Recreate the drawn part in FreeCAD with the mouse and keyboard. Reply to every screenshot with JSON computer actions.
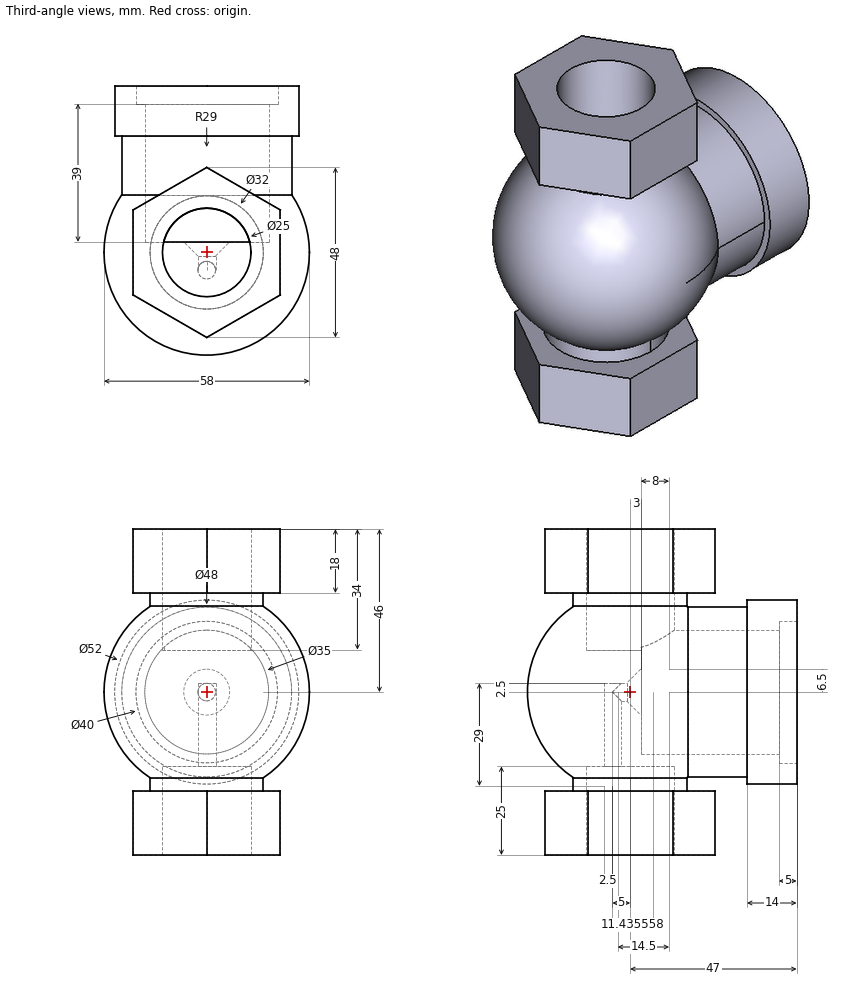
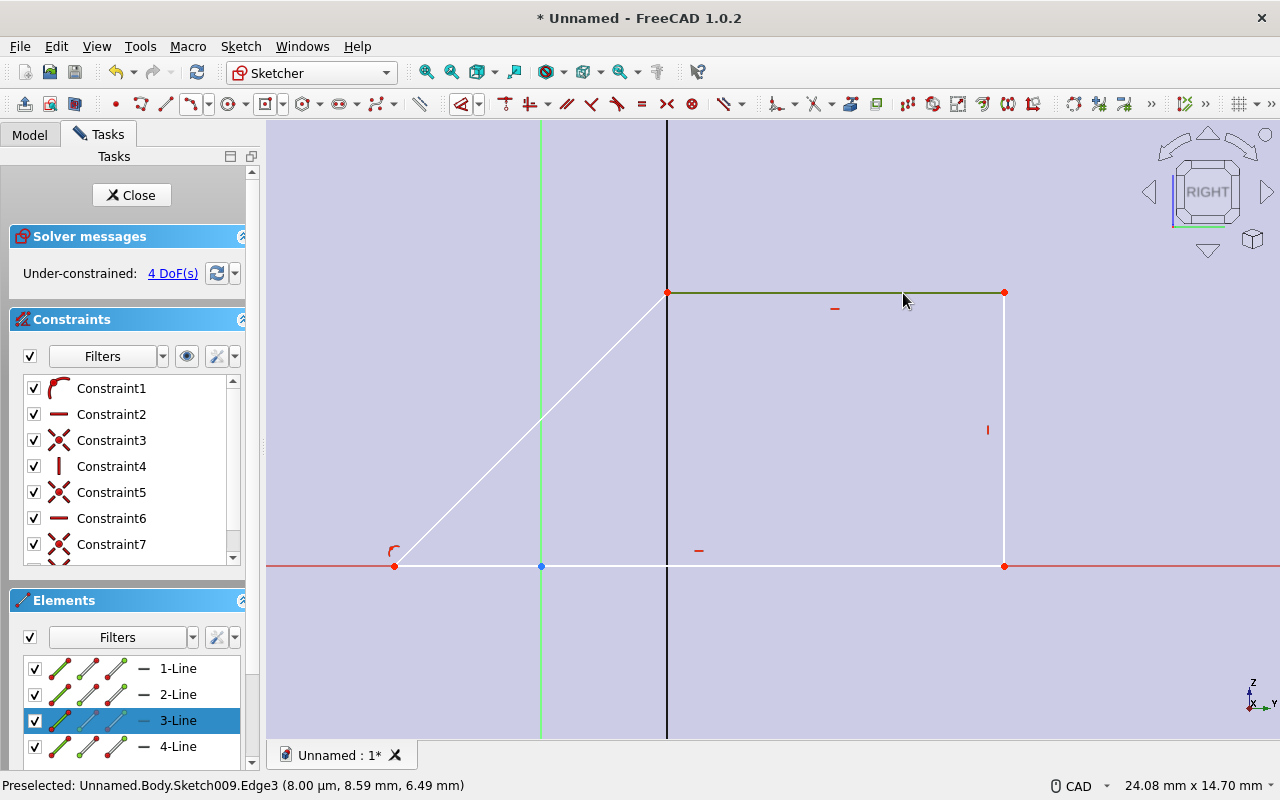
{"action": "left_click", "coordinate": [478, 104]}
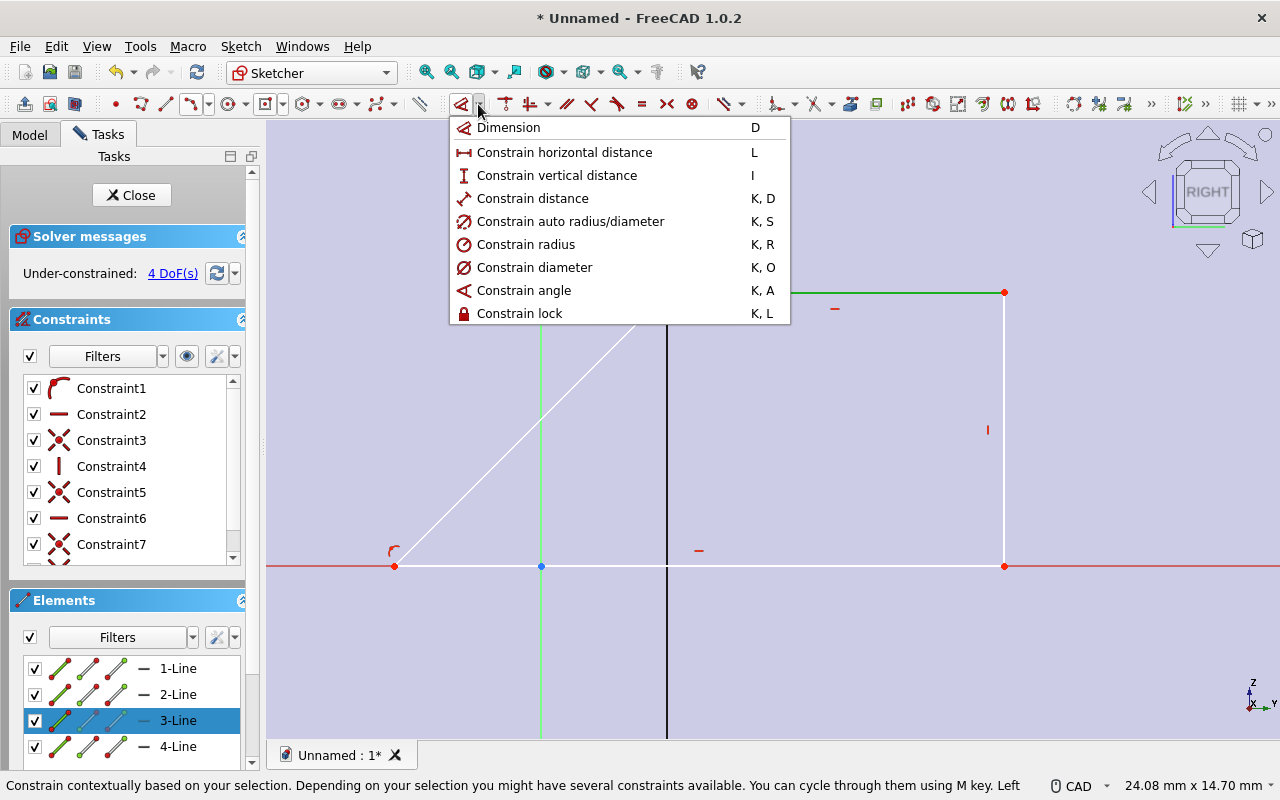
{"action": "left_click", "coordinate": [620, 152]}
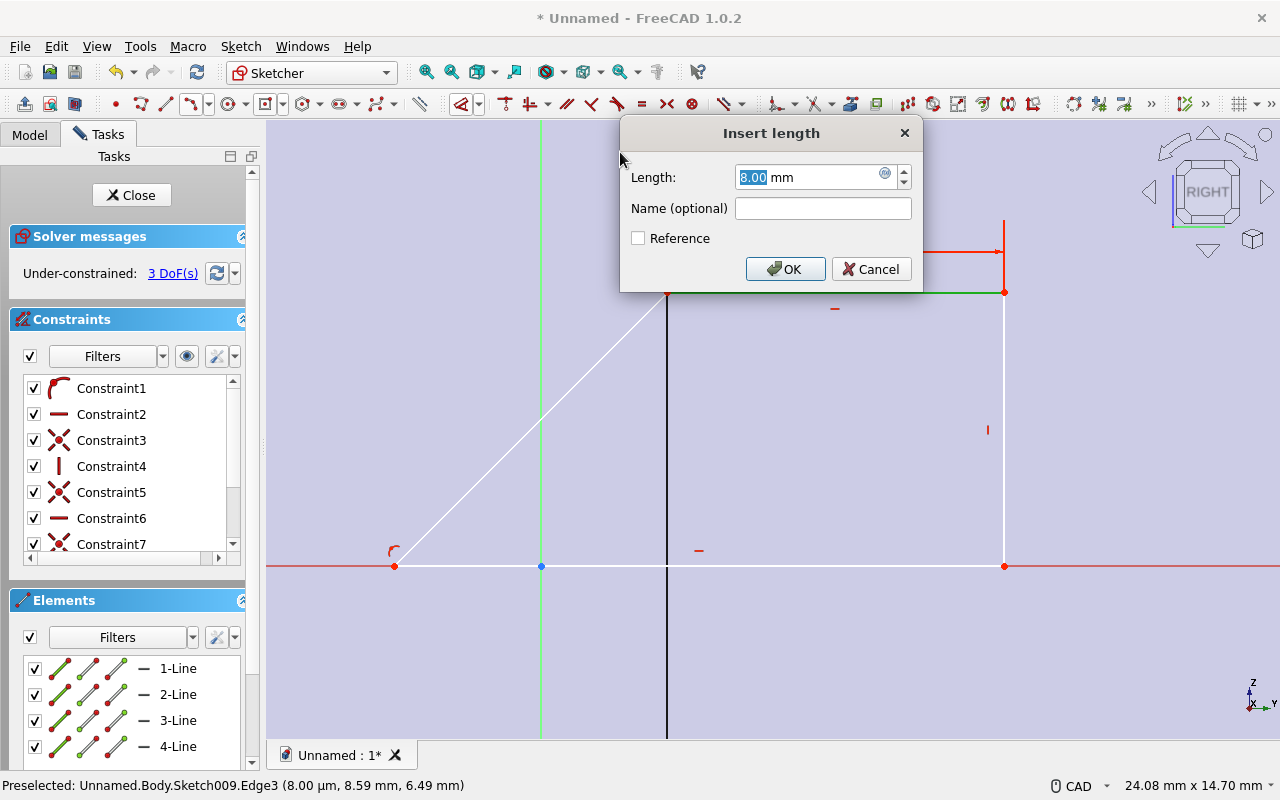
{"action": "type", "text": "8"}
{"action": "key", "text": "Return"}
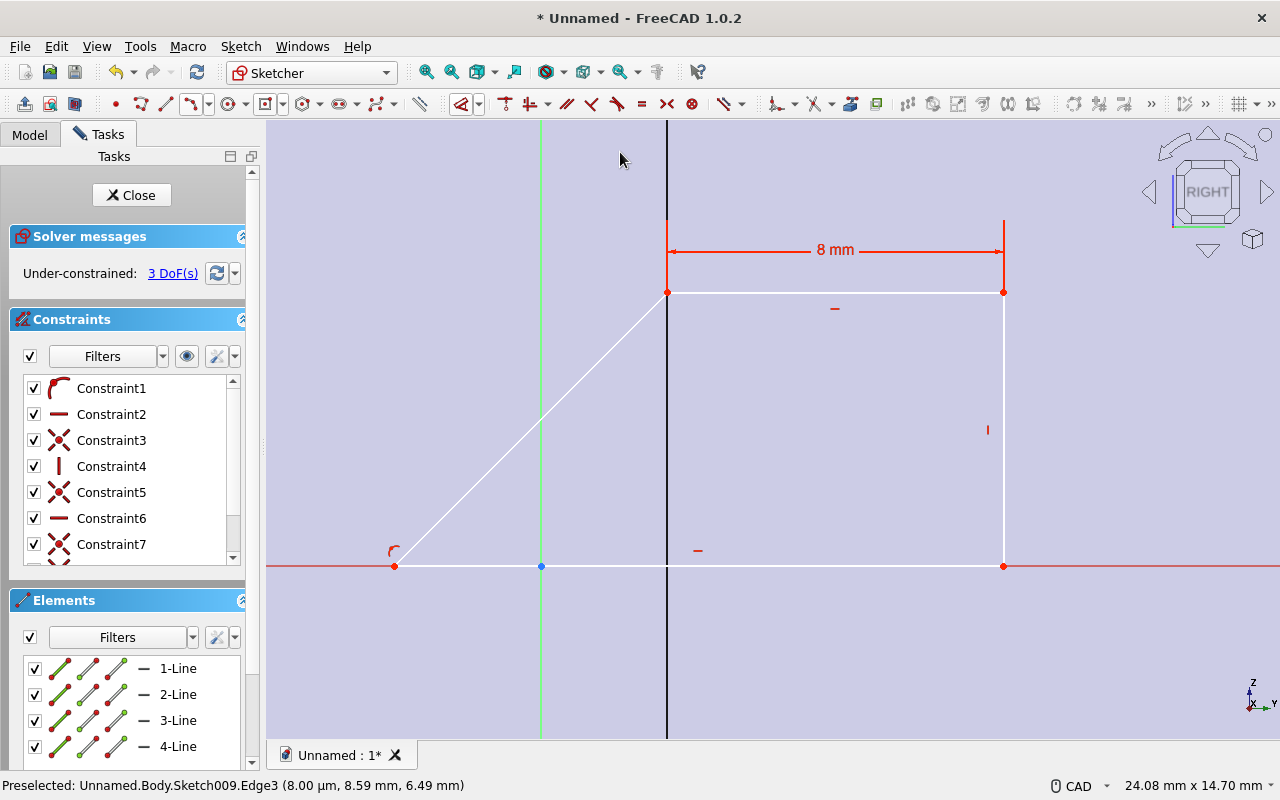
{"action": "left_click", "coordinate": [667, 293]}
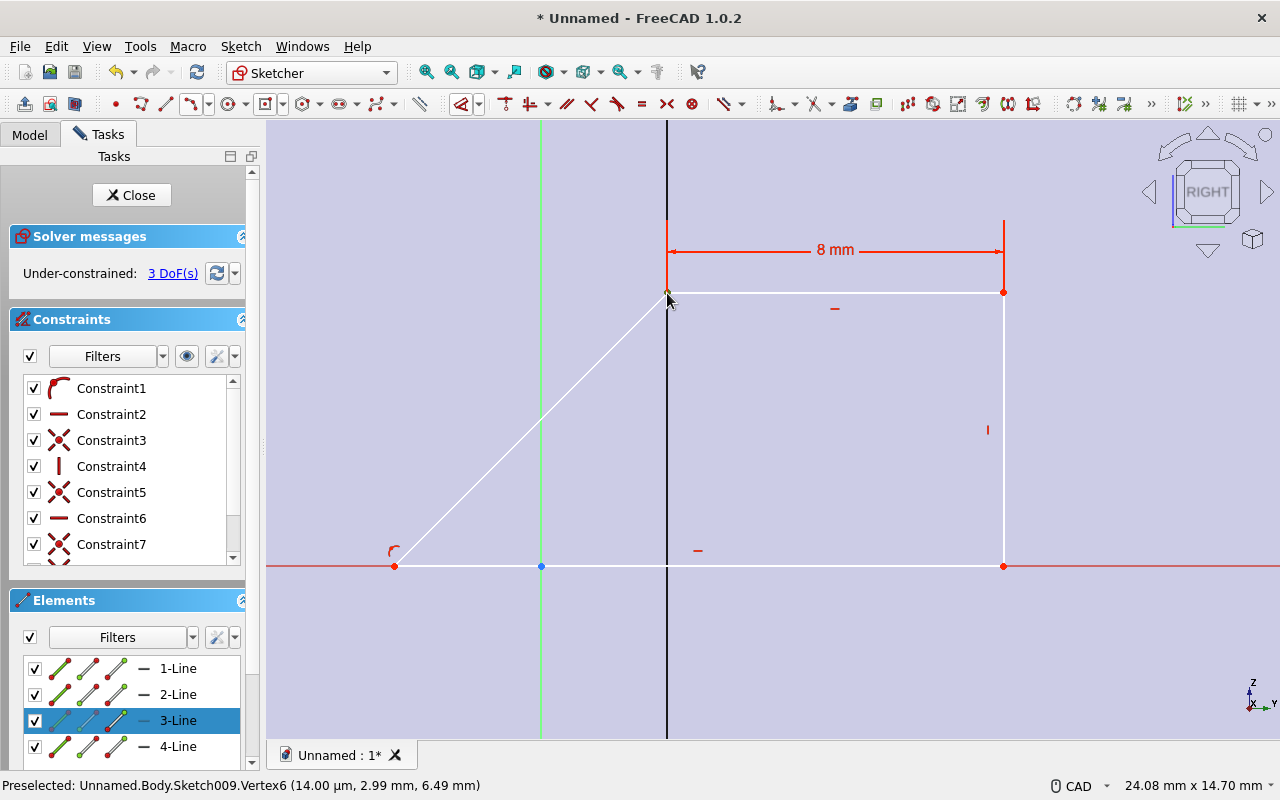
{"action": "key", "text": "l"}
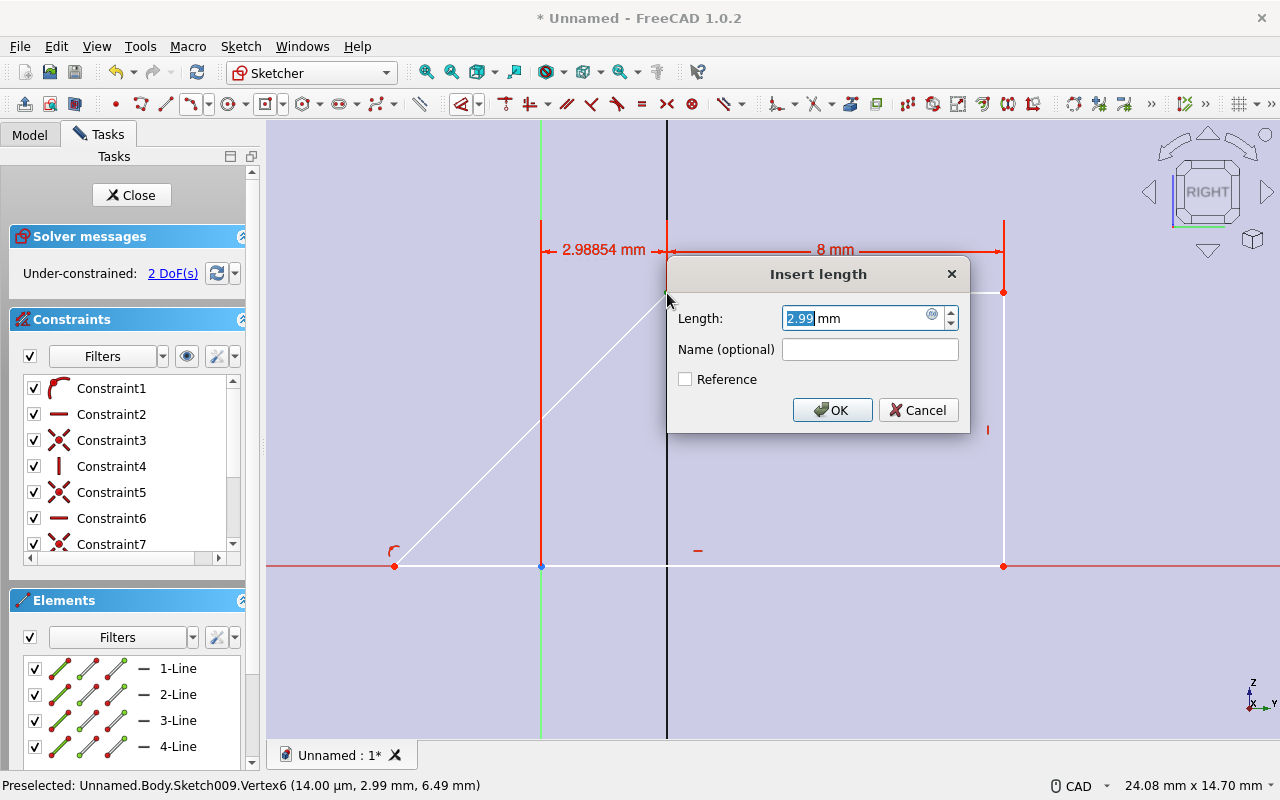
{"action": "type", "text": "3"}
{"action": "key", "text": "Return"}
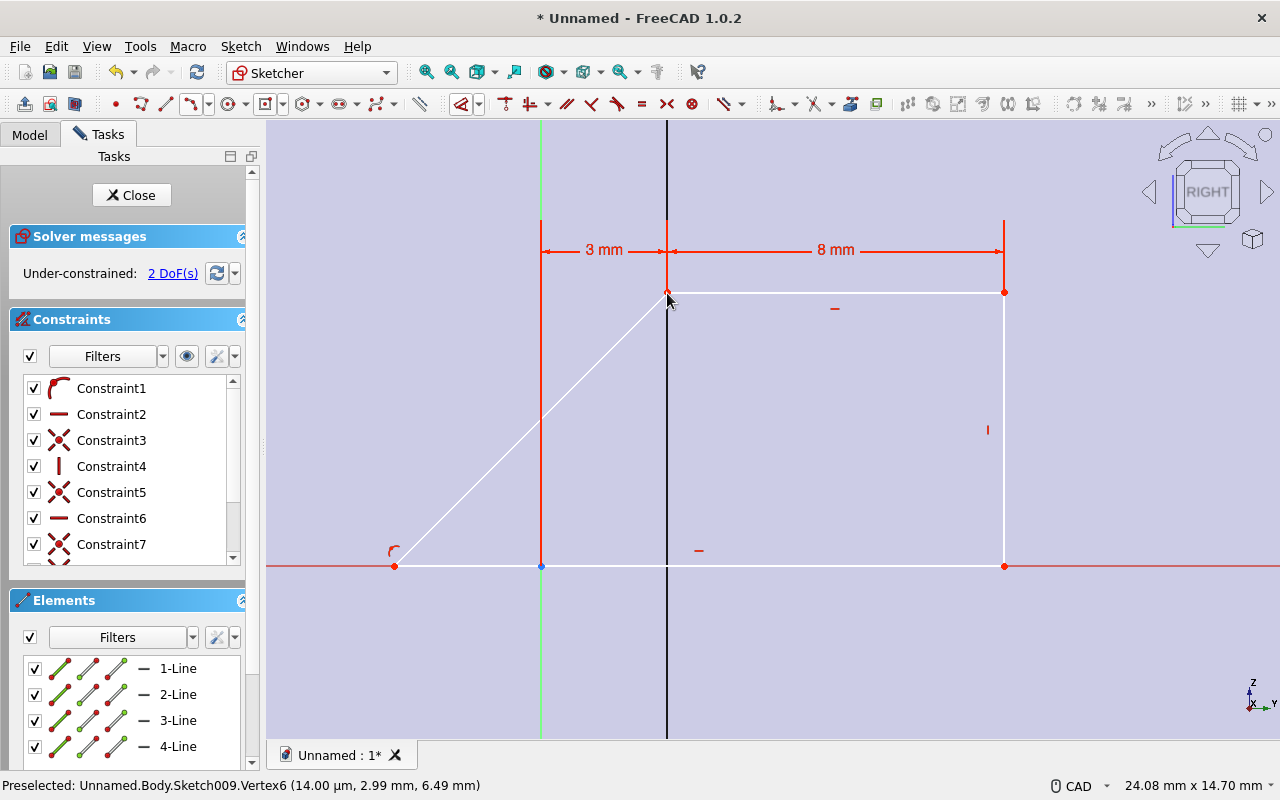
{"action": "left_click", "coordinate": [1004, 484]}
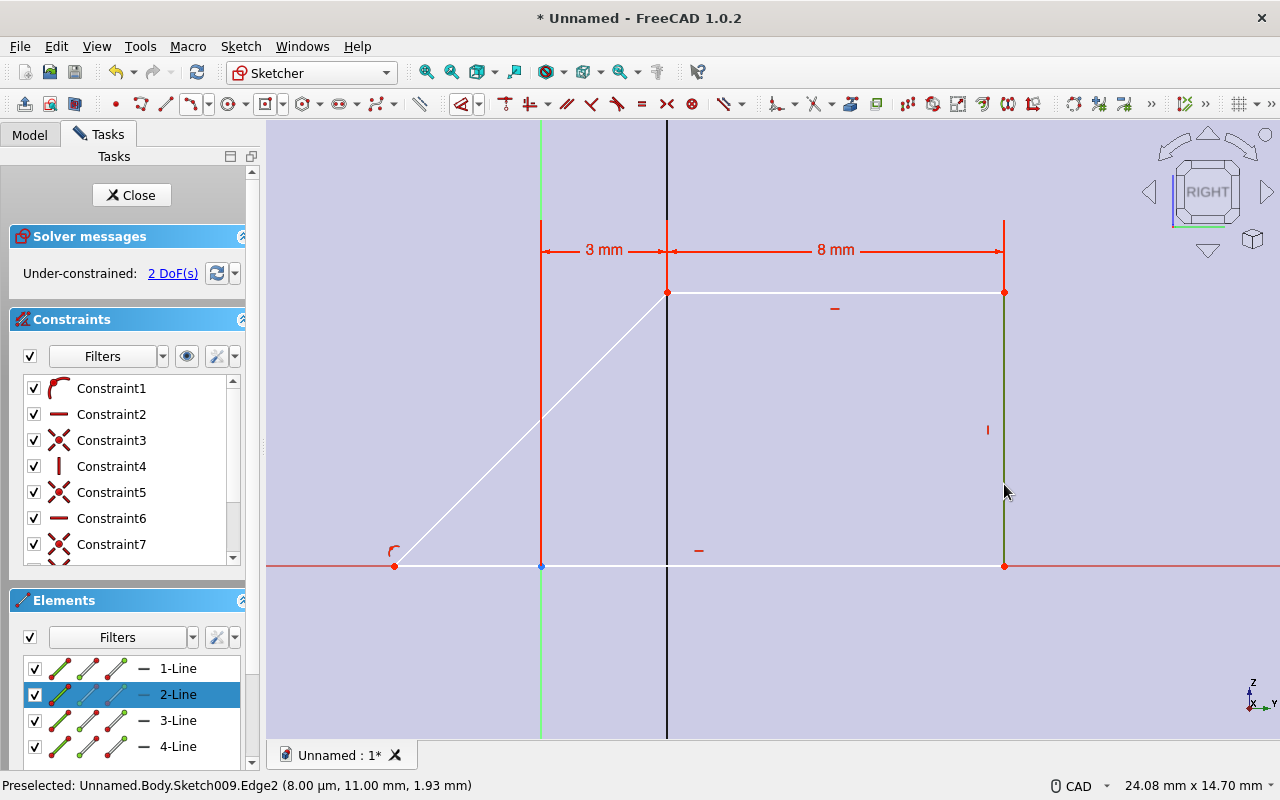
{"action": "key", "text": "i"}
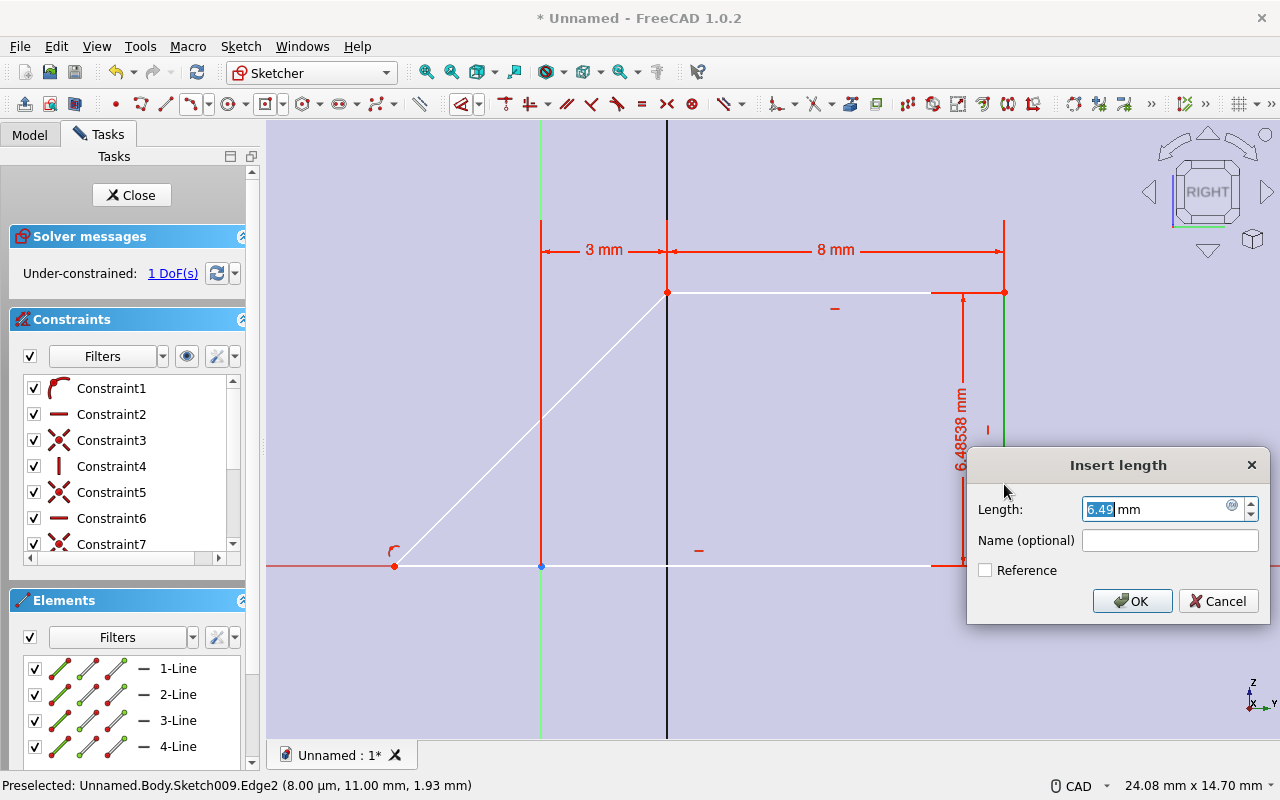
{"action": "type", "text": "6.5"}
{"action": "key", "text": "Return"}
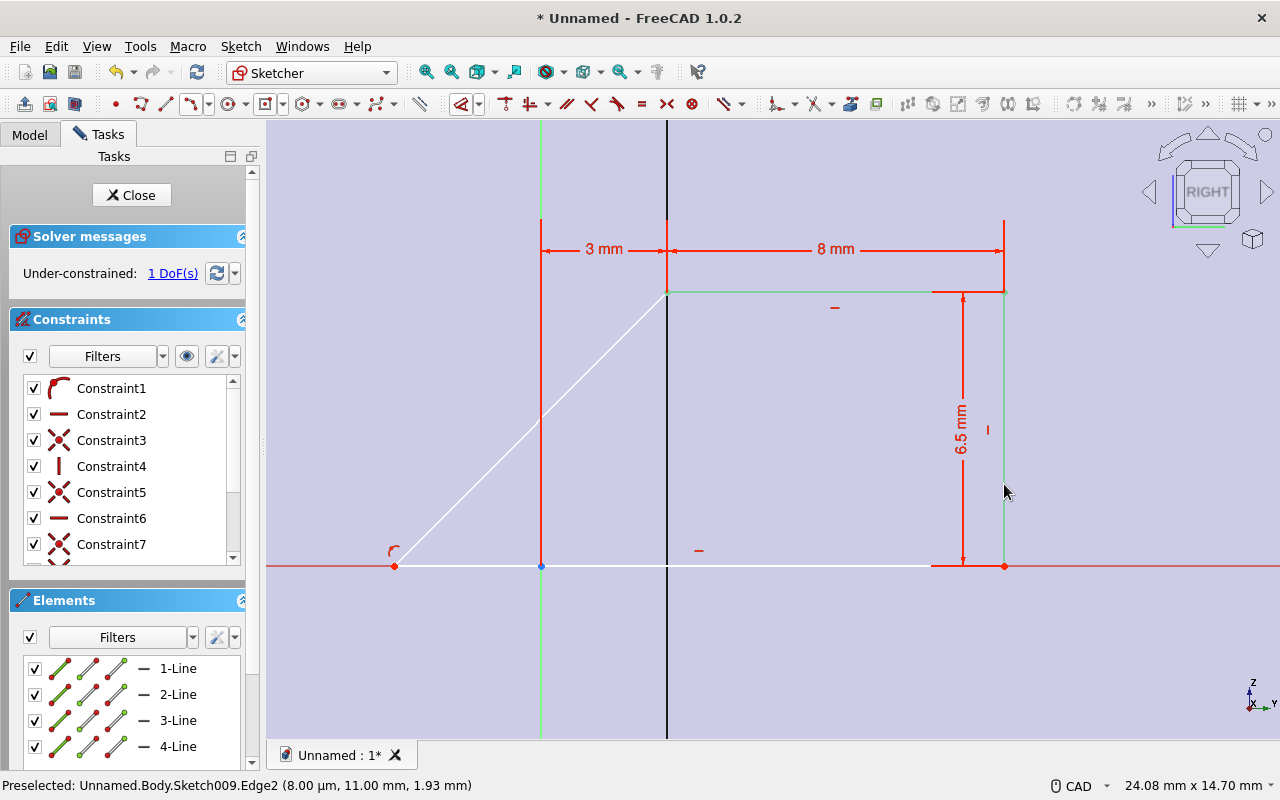
{"action": "left_click", "coordinate": [577, 566]}